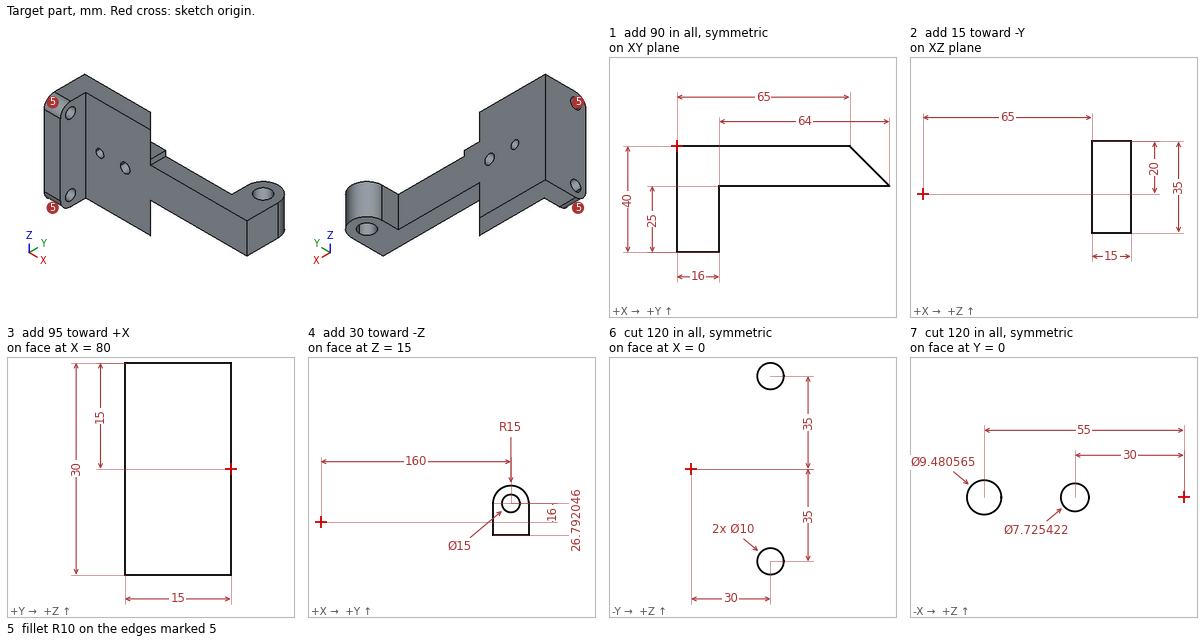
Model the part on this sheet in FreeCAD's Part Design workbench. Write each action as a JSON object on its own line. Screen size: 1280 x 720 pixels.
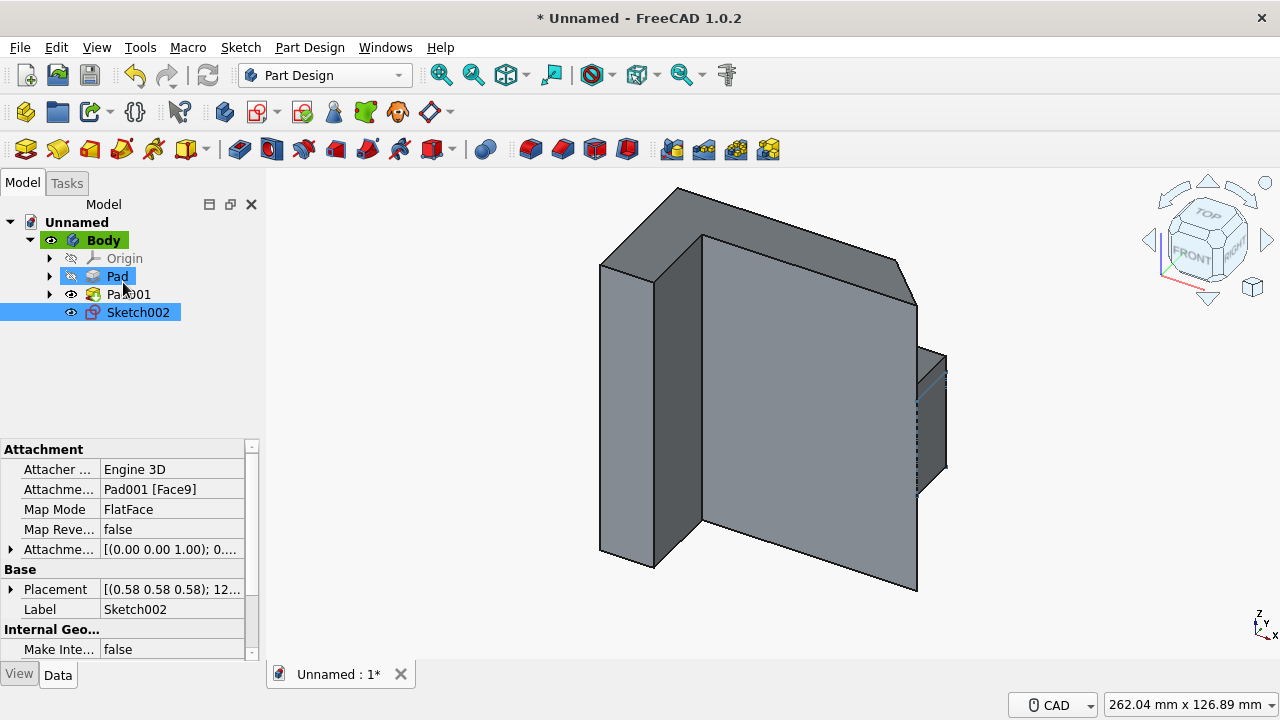
{"action": "left_click", "coordinate": [26, 150]}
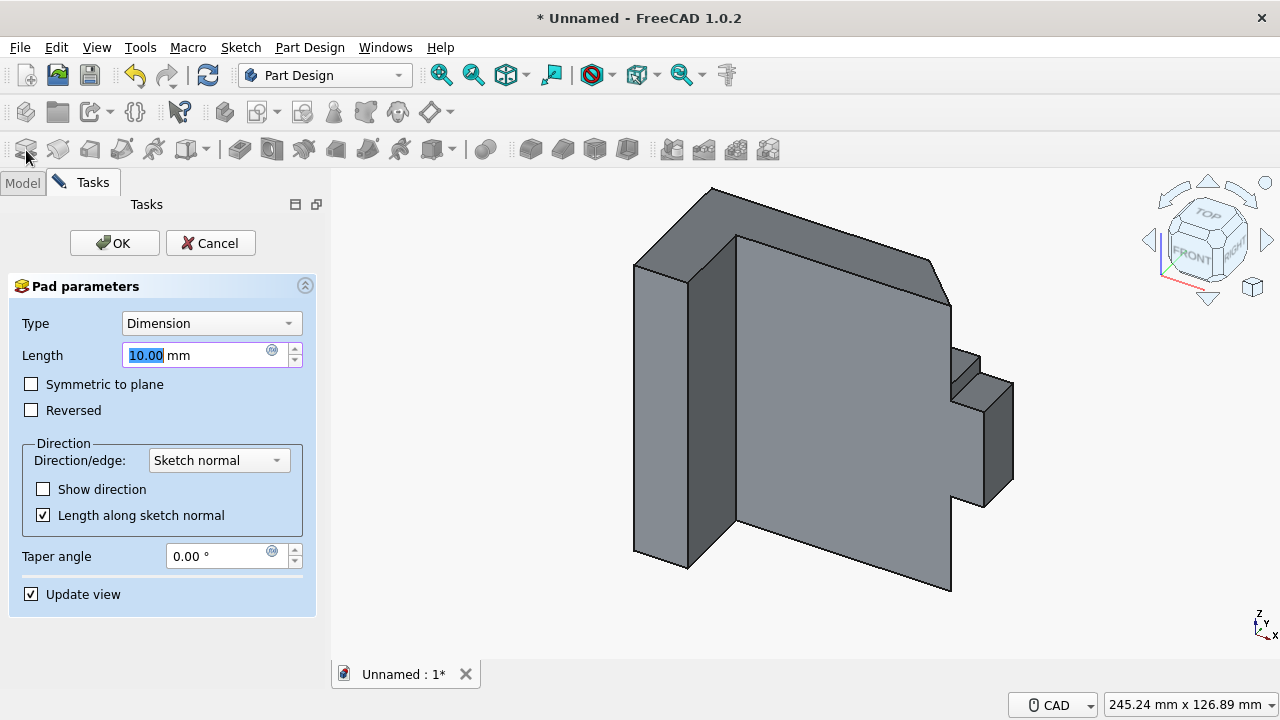
{"action": "type", "text": "95"}
{"action": "key", "text": "Tab"}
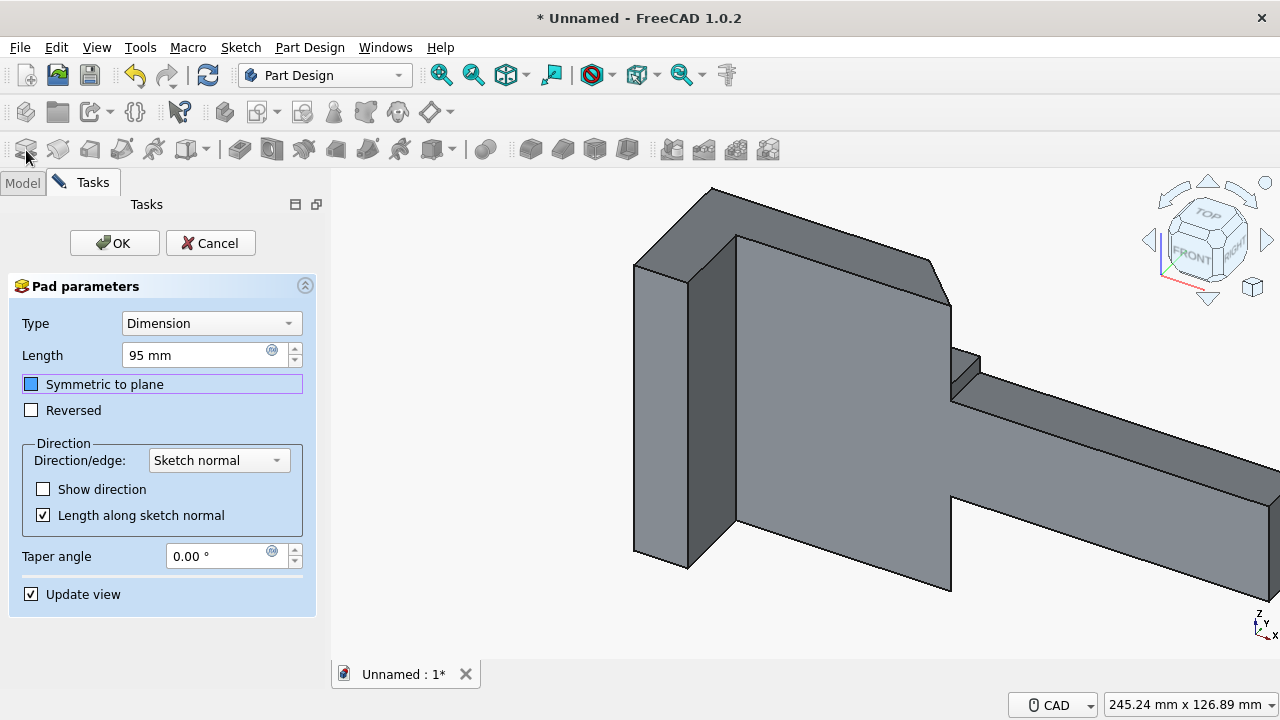
{"action": "left_click", "coordinate": [115, 243]}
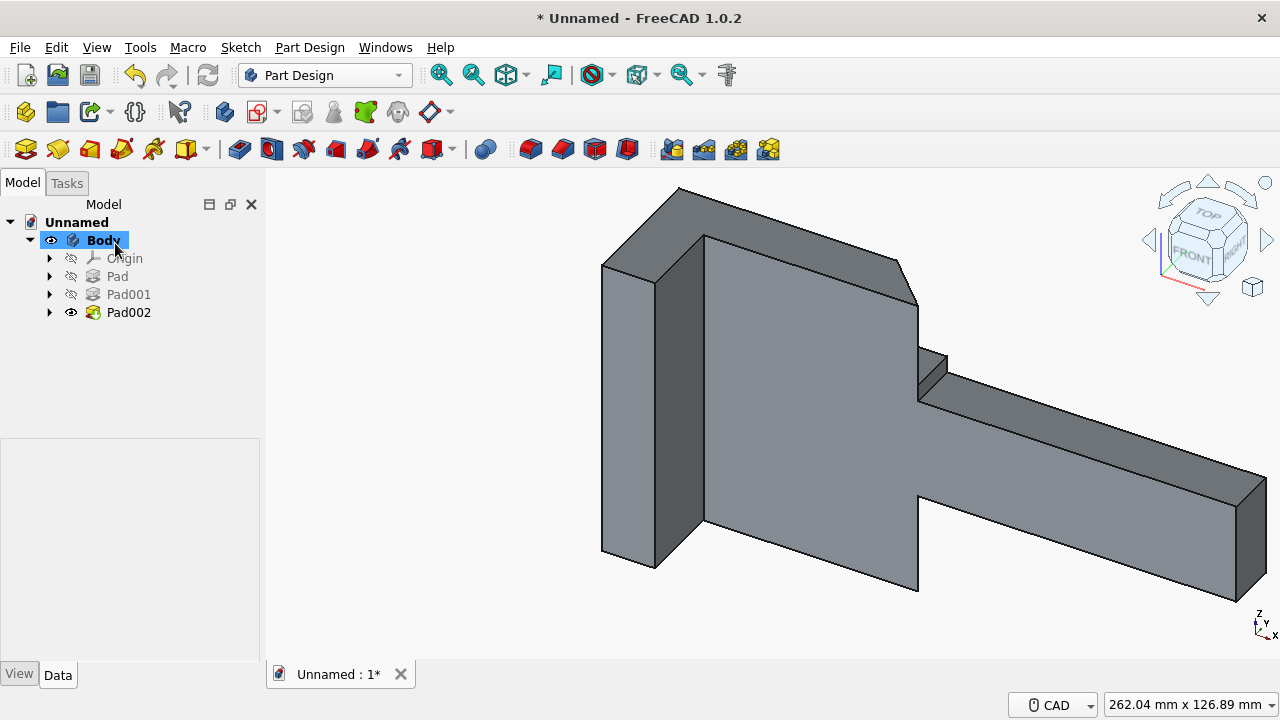
{"action": "left_click", "coordinate": [442, 76]}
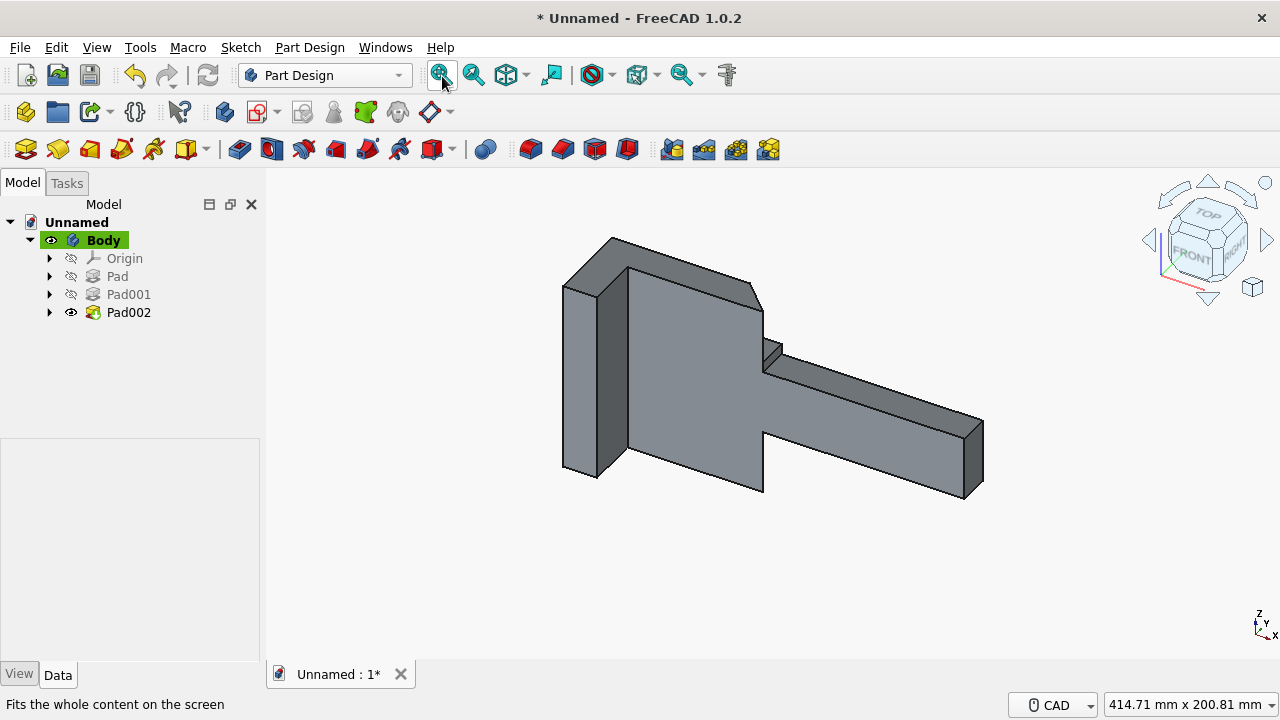
{"action": "left_click", "coordinate": [930, 414]}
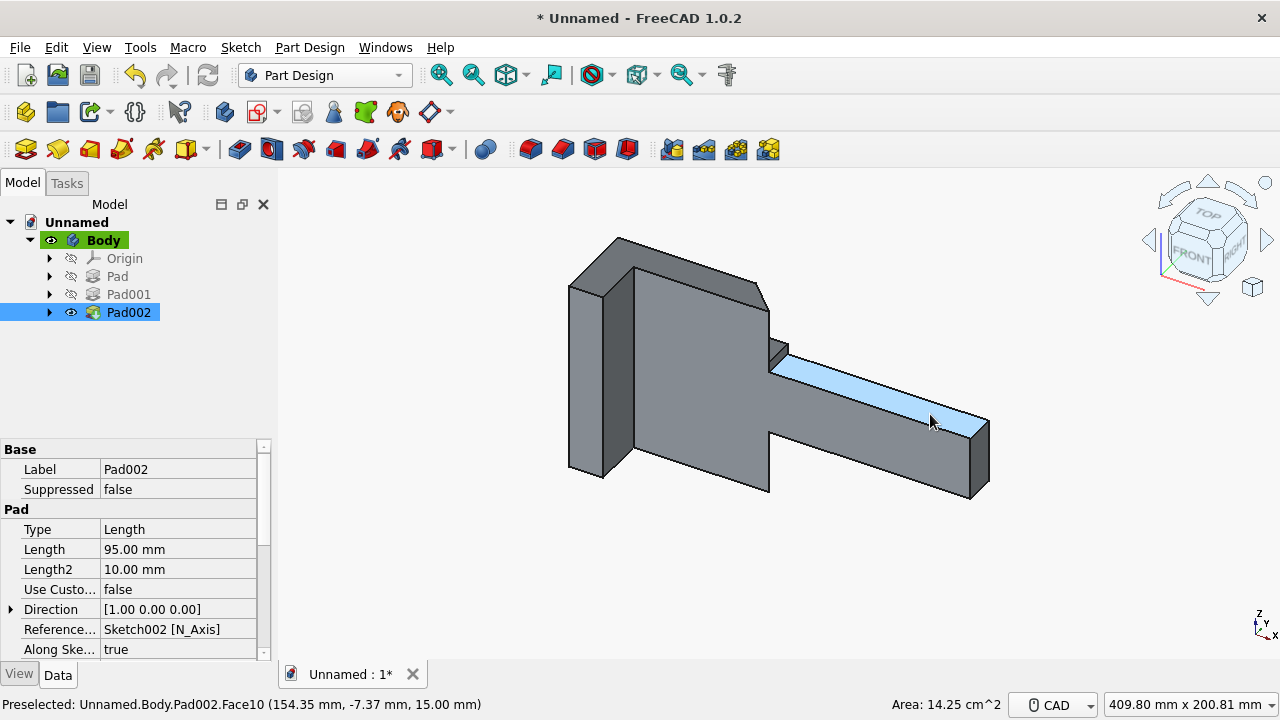
{"action": "left_click", "coordinate": [258, 112]}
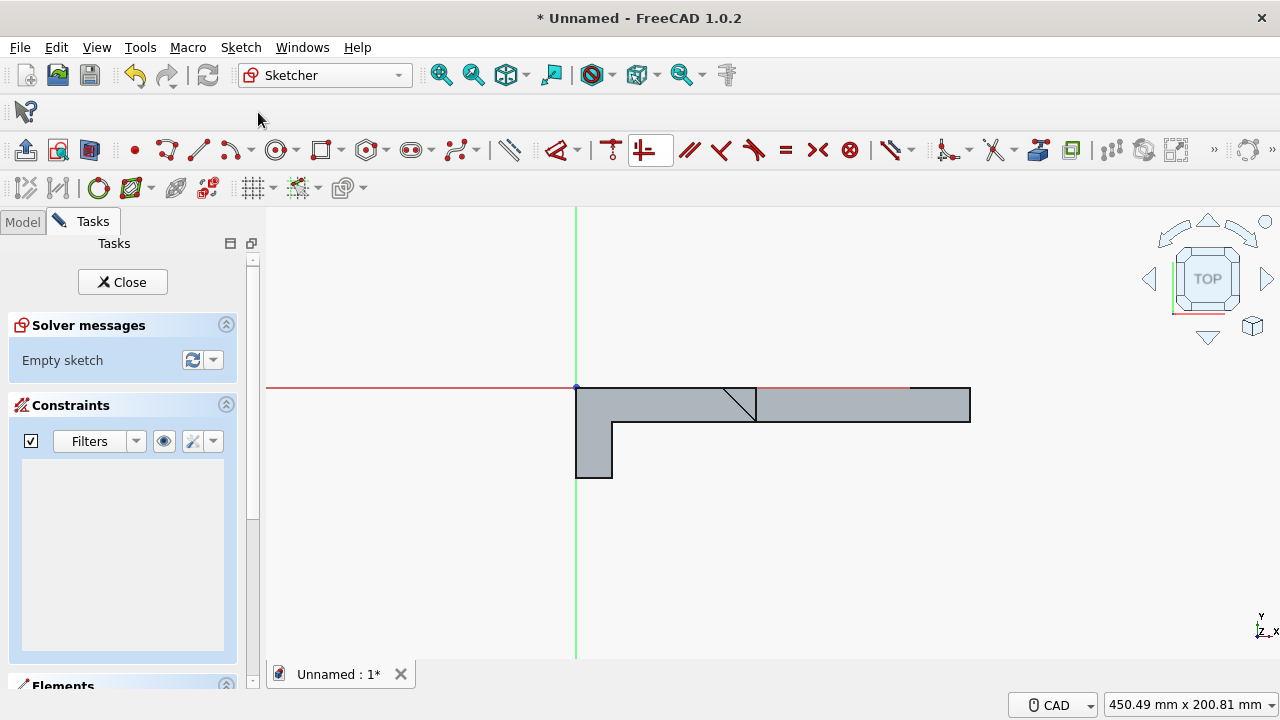
{"action": "scroll", "coordinate": [1071, 326], "scroll_direction": "up", "scroll_amount": 5}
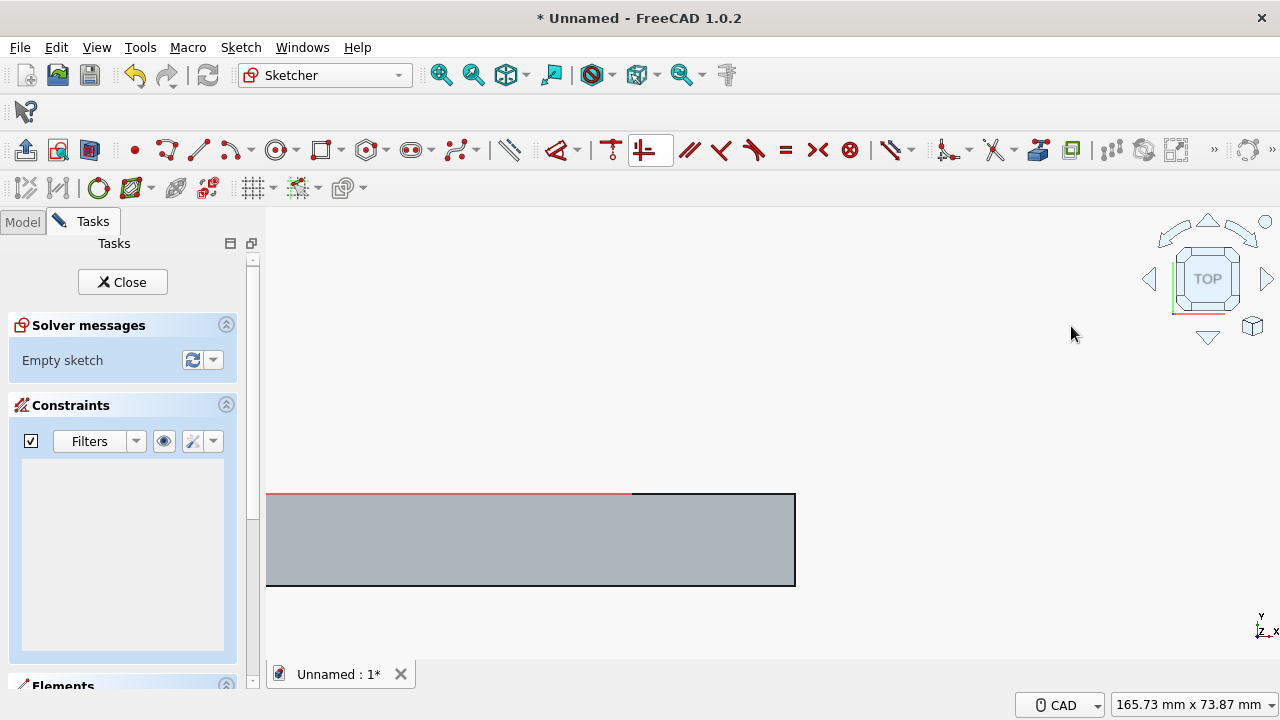
{"action": "left_click", "coordinate": [168, 150]}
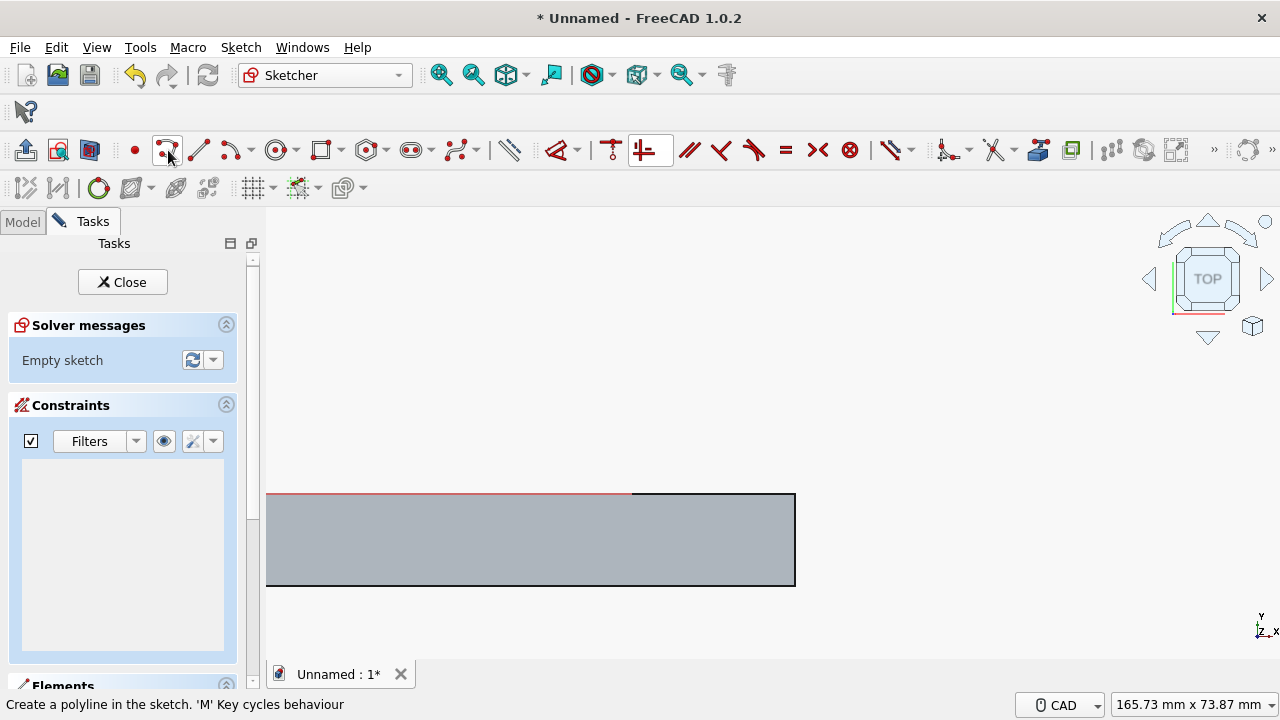
{"action": "left_click", "coordinate": [611, 396]}
{"action": "left_click", "coordinate": [611, 560]}
{"action": "left_click", "coordinate": [795, 560]}
{"action": "left_click", "coordinate": [795, 396]}
{"action": "right_click", "coordinate": [795, 396]}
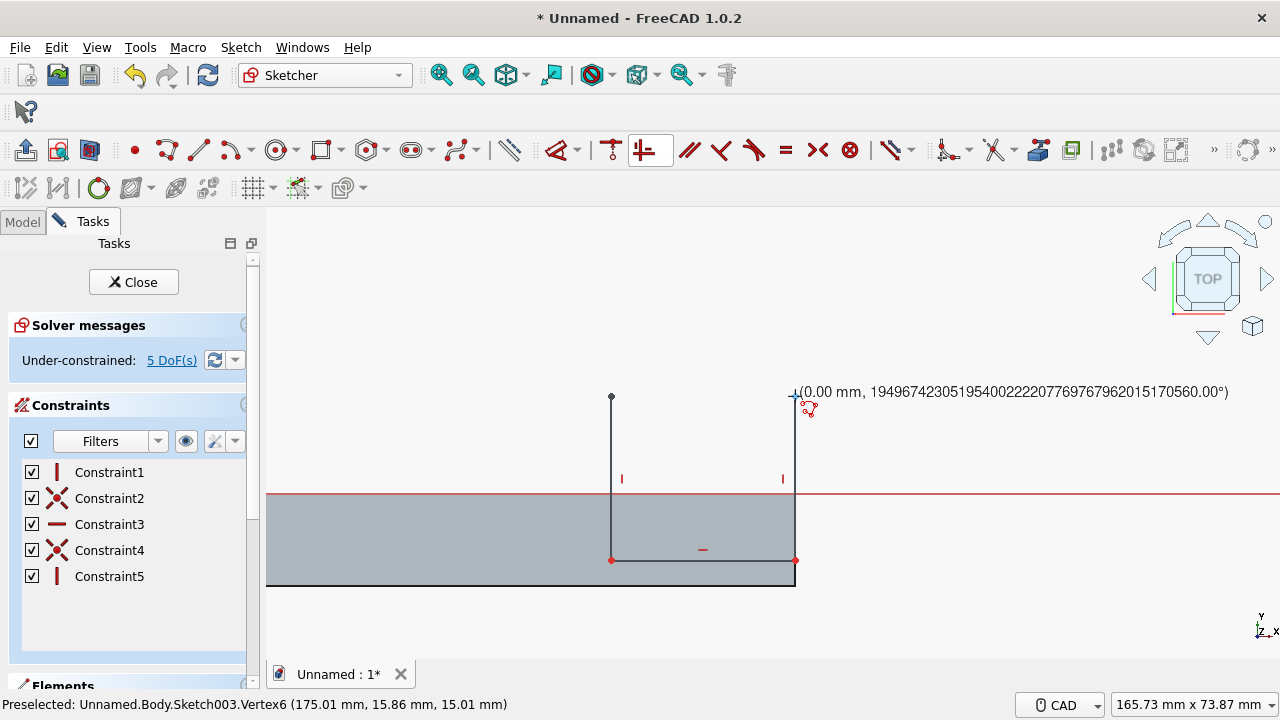
{"action": "key", "text": "g 3 a"}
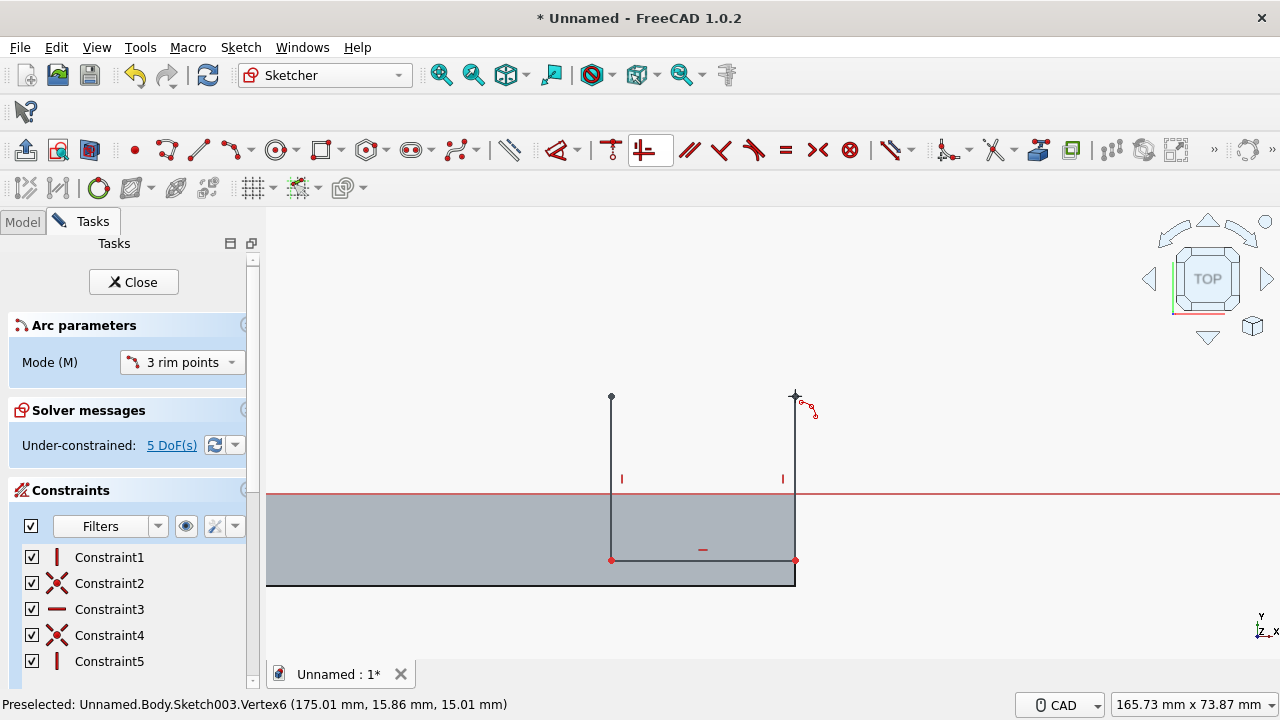
{"action": "left_click", "coordinate": [795, 397]}
{"action": "left_click", "coordinate": [611, 397]}
{"action": "left_click", "coordinate": [703, 304]}